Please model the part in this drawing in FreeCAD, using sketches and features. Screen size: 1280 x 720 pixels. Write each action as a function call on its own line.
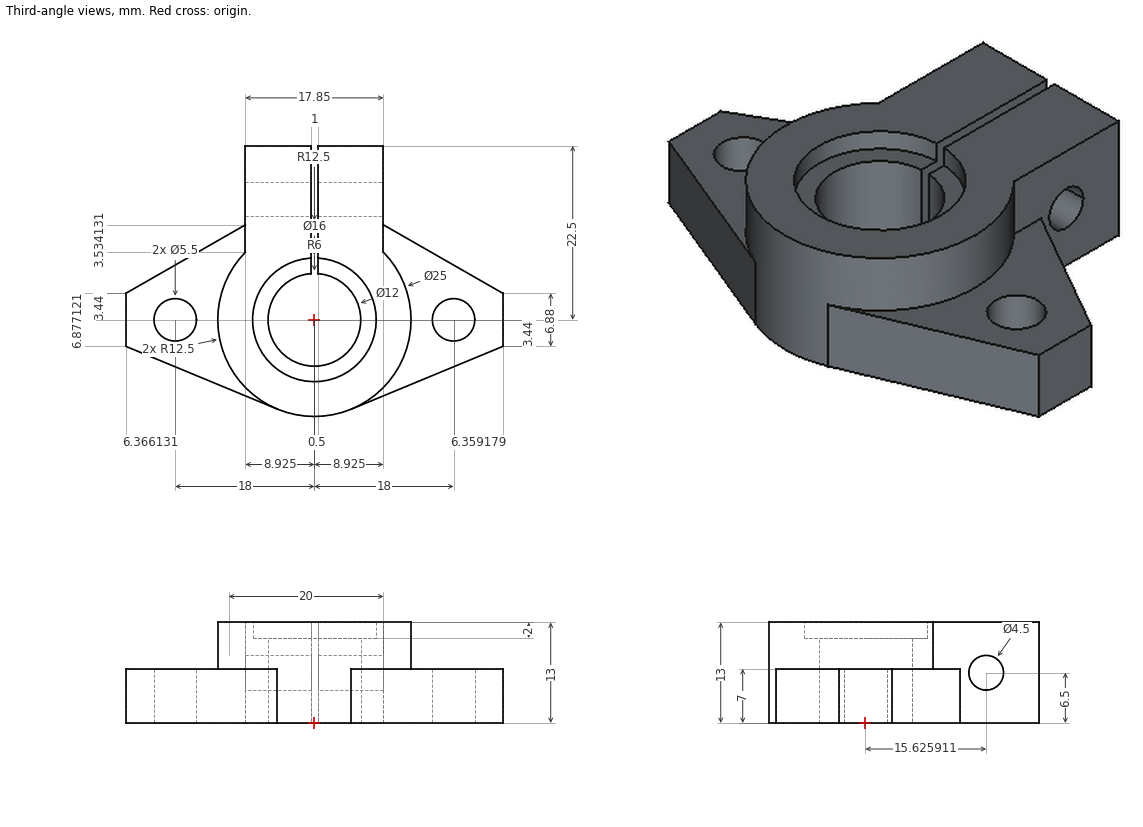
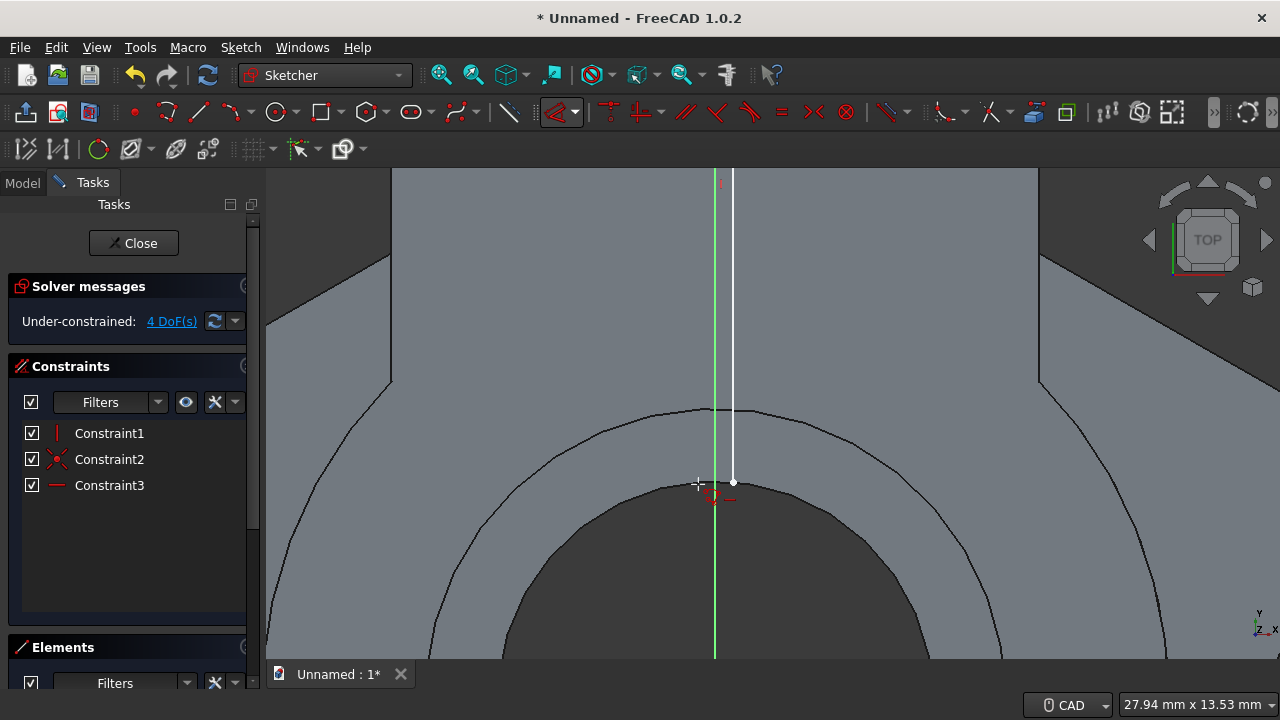
click(697, 482)
right_click(697, 482)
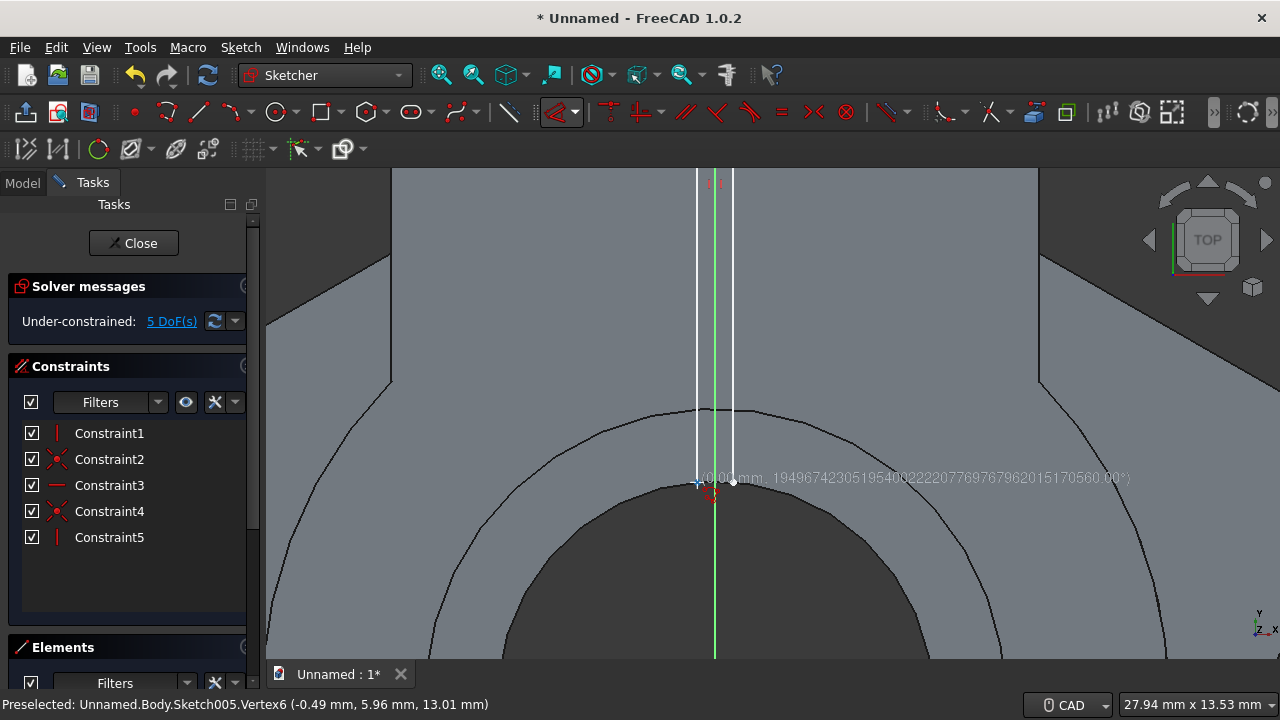
click(232, 112)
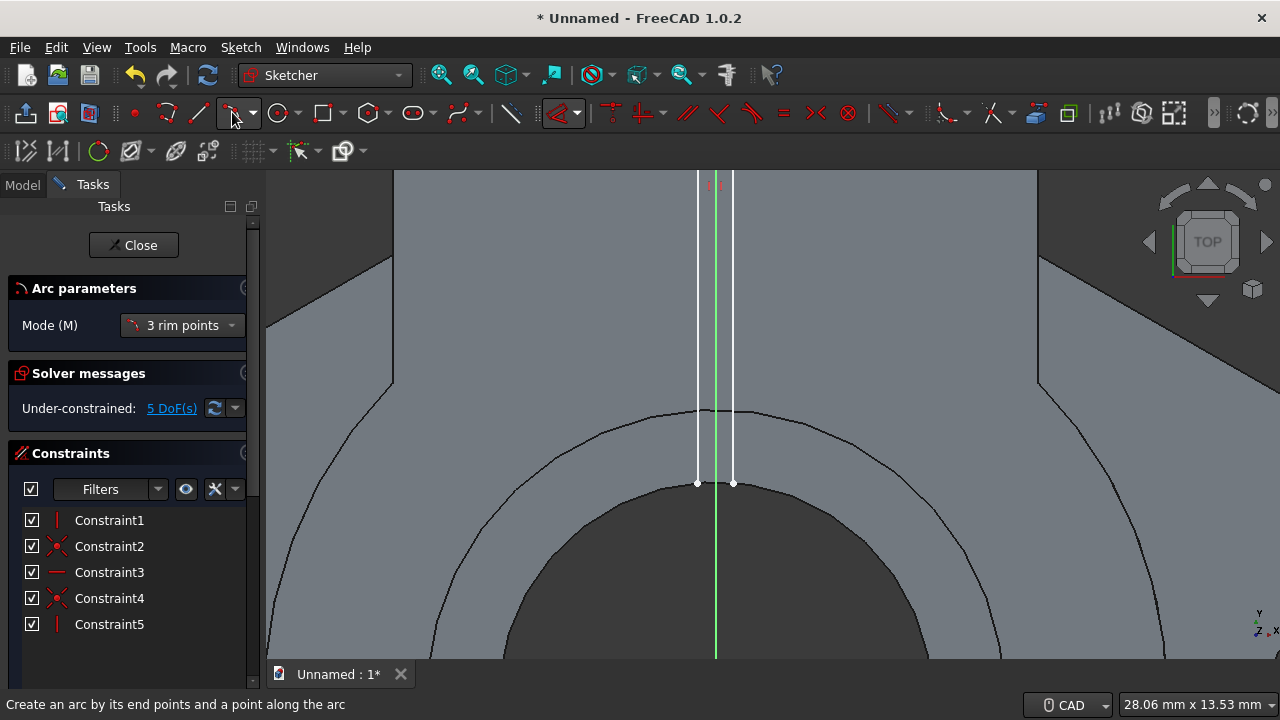
click(698, 484)
click(733, 484)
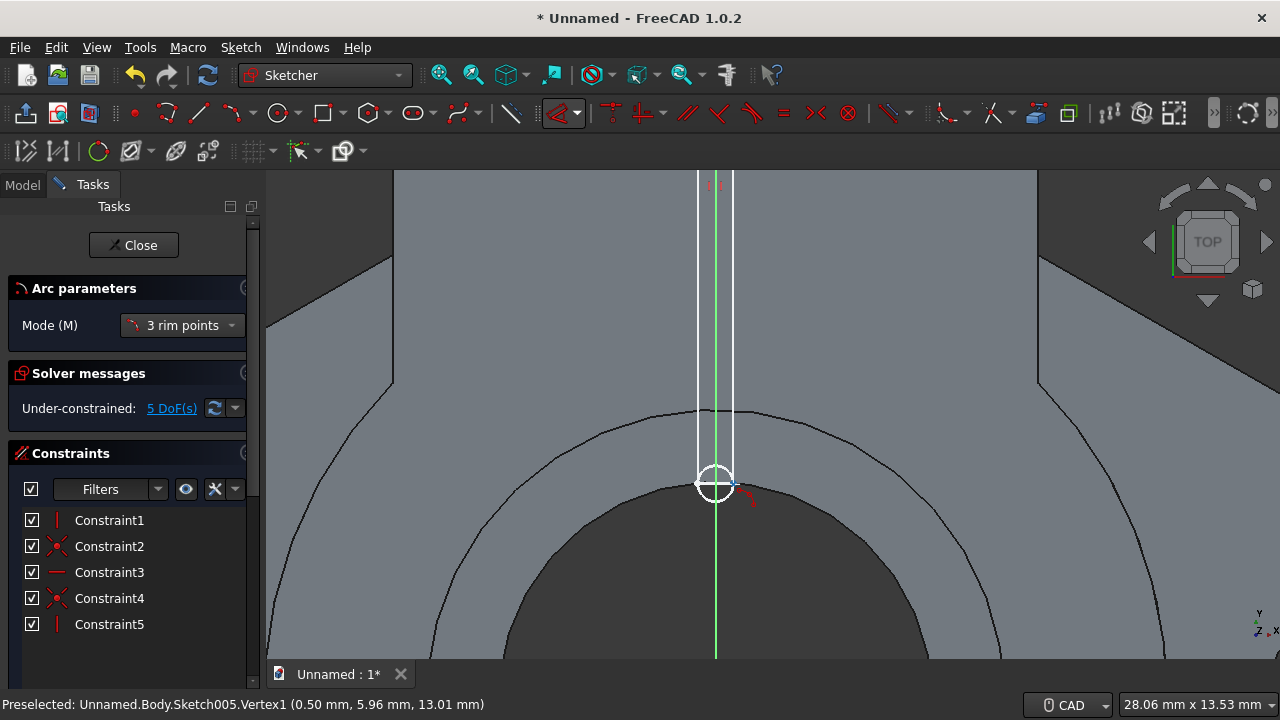
scroll(719, 482, up, 16)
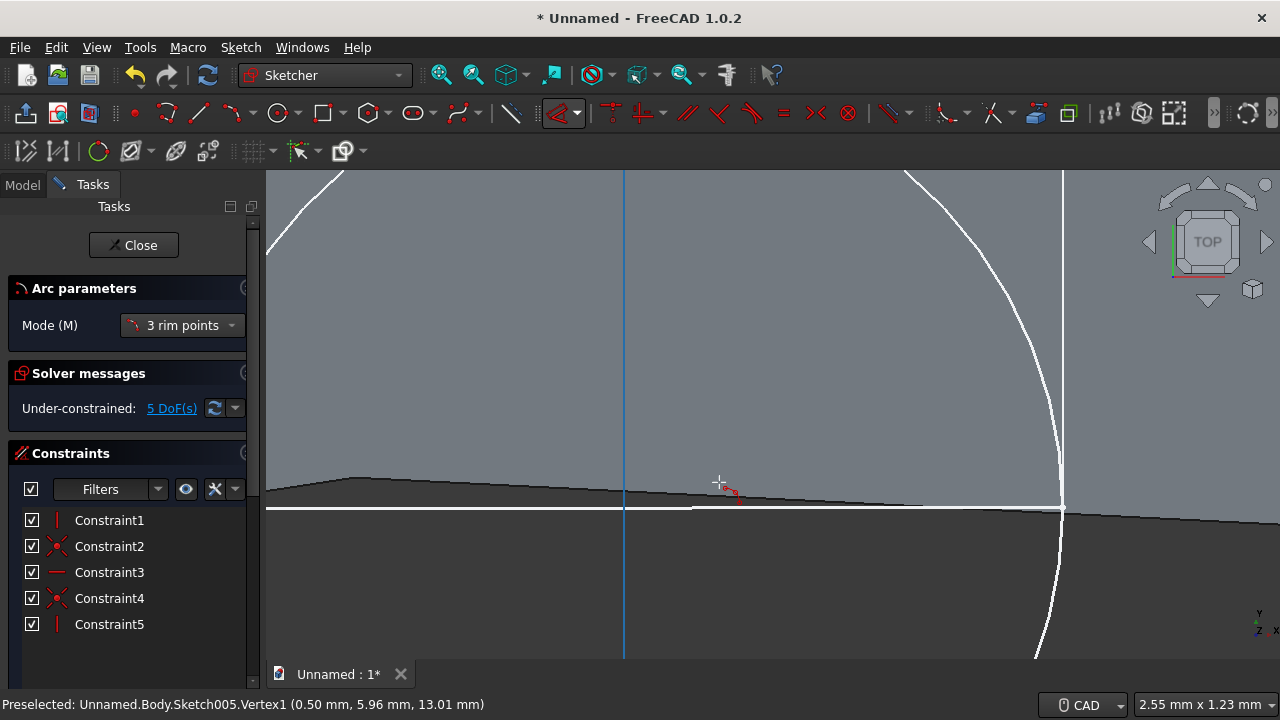
click(713, 472)
key(Escape)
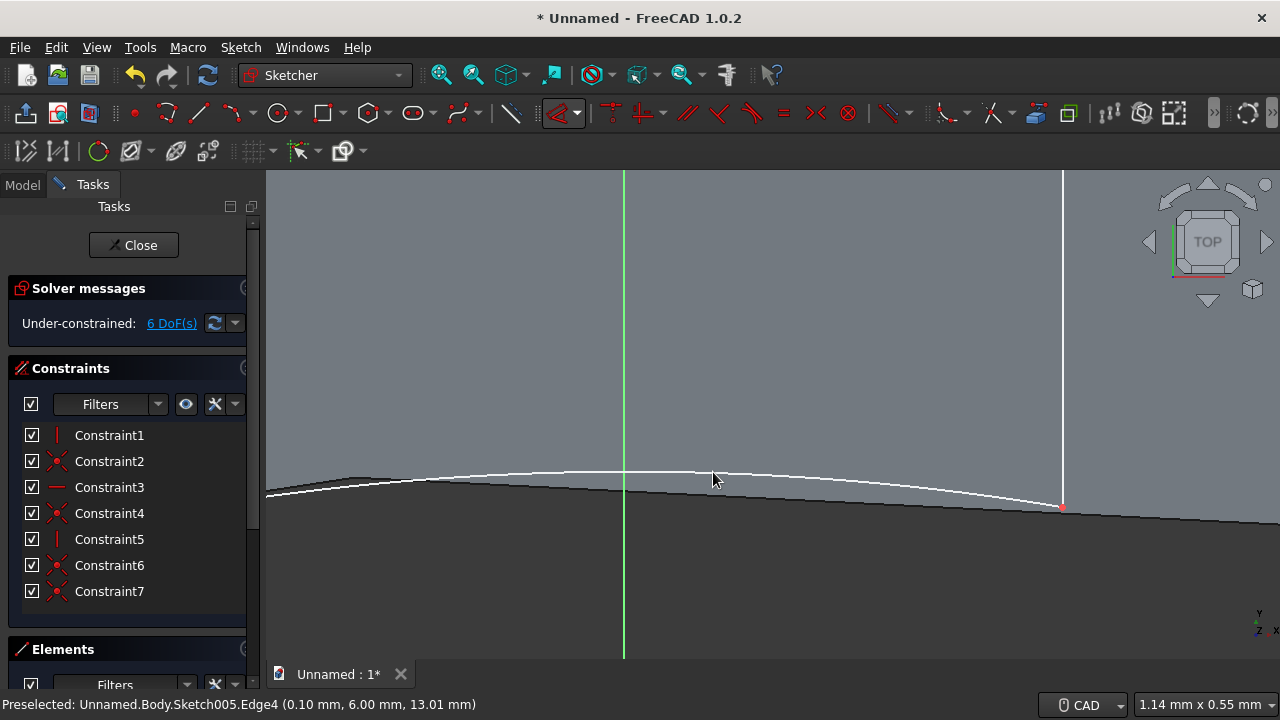
scroll(704, 414, down, 15)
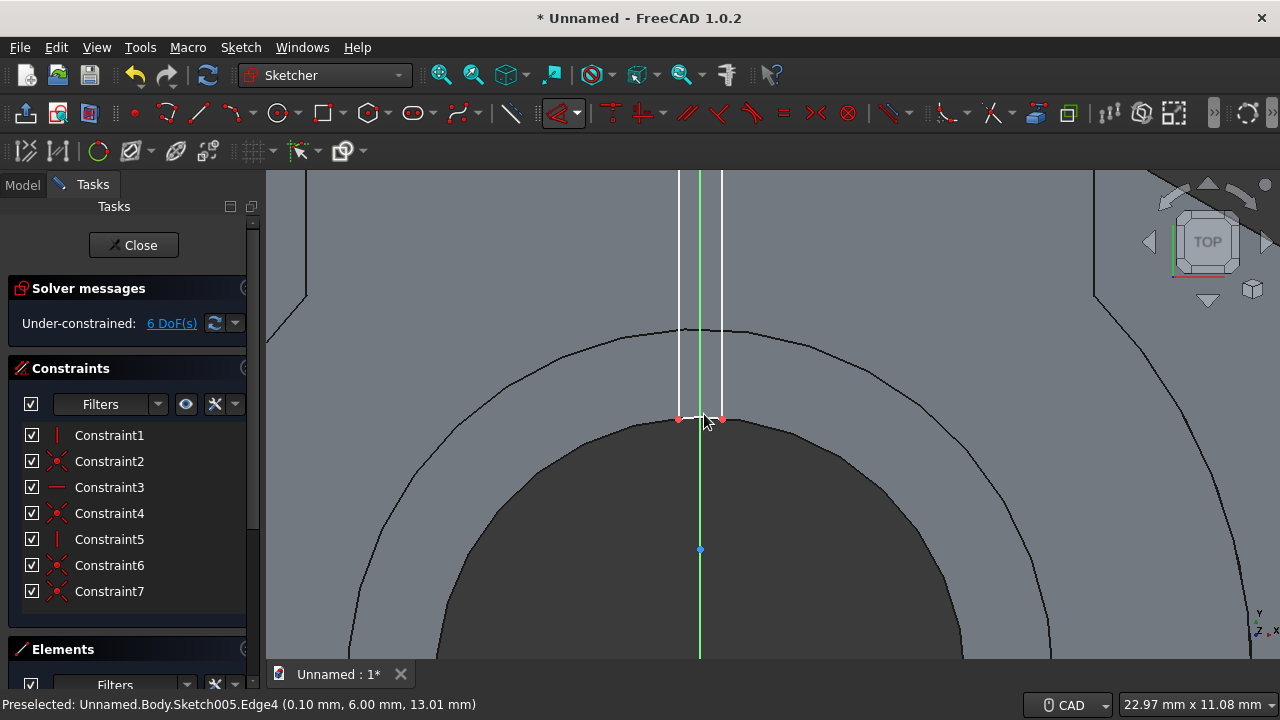
scroll(706, 513, down, 6)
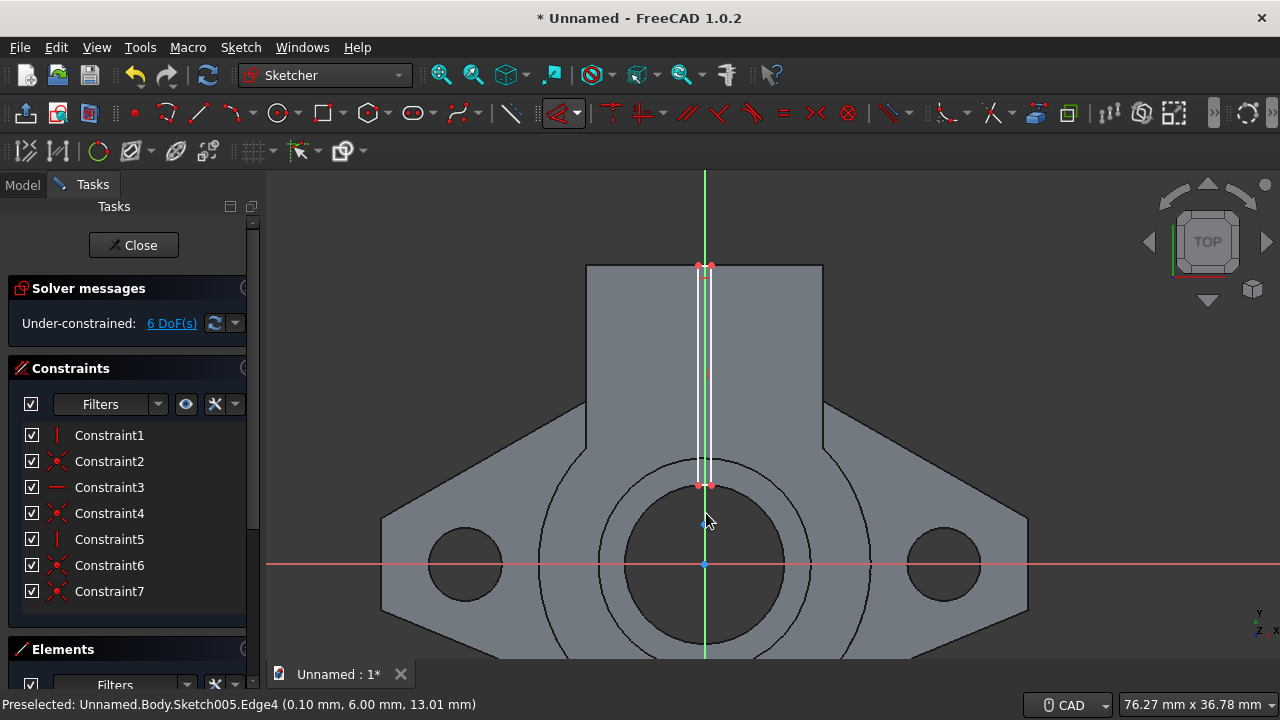
drag(695, 515, 715, 574)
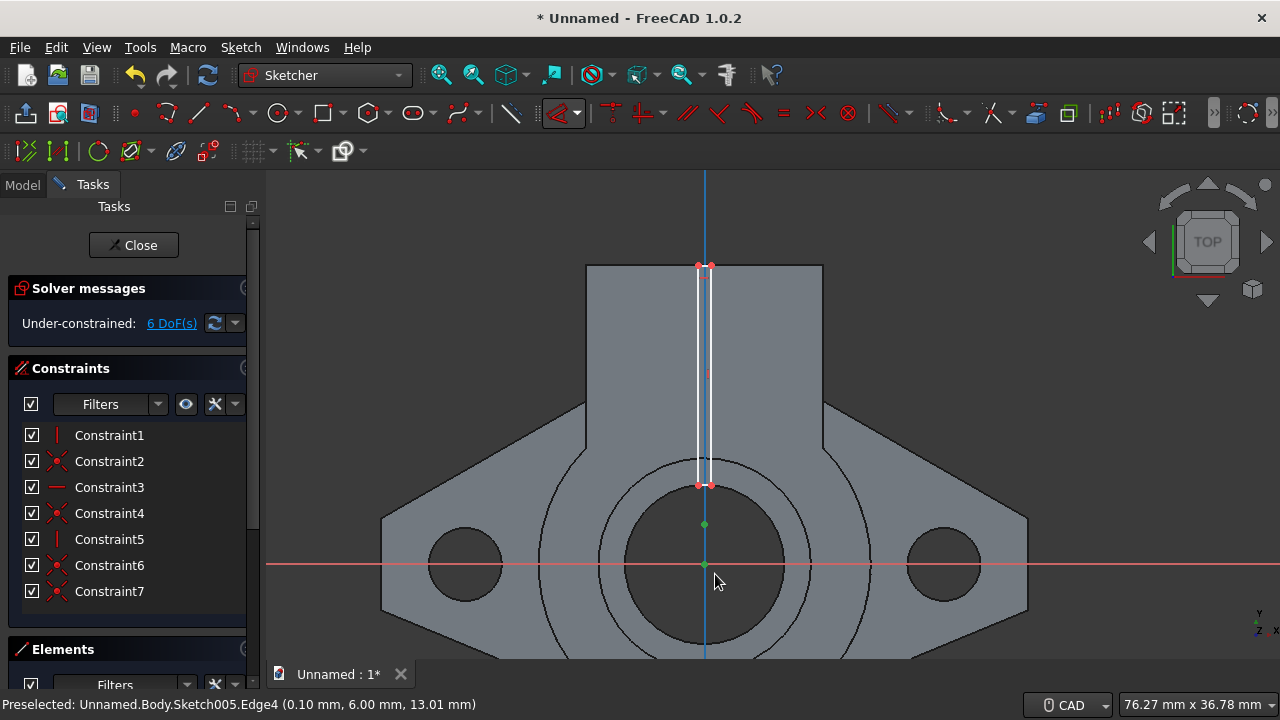
click(612, 114)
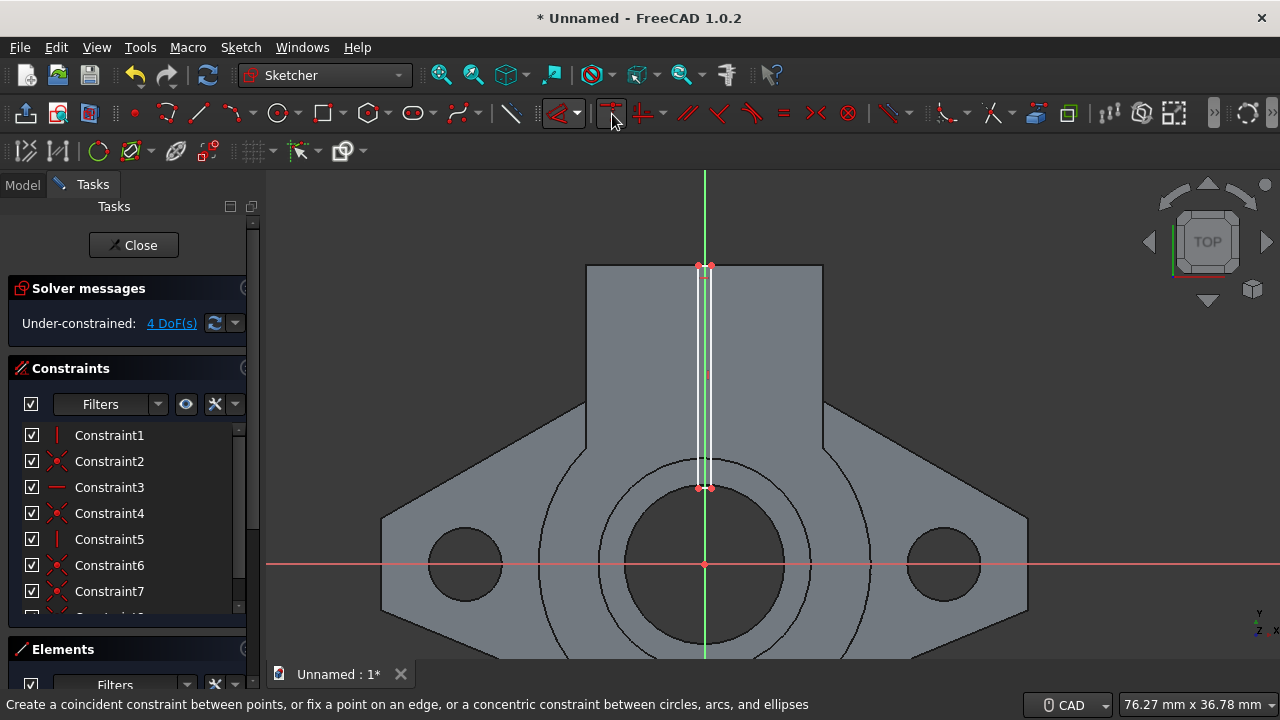
scroll(705, 488, up, 4)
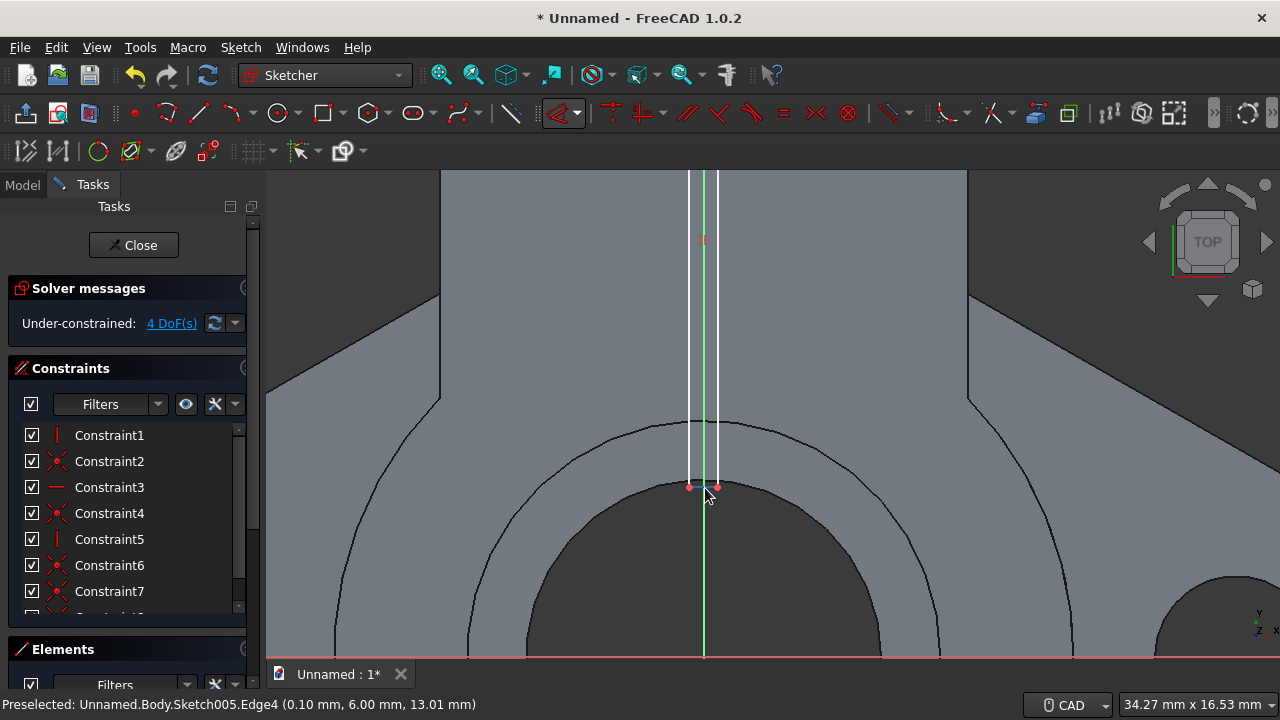
click(704, 487)